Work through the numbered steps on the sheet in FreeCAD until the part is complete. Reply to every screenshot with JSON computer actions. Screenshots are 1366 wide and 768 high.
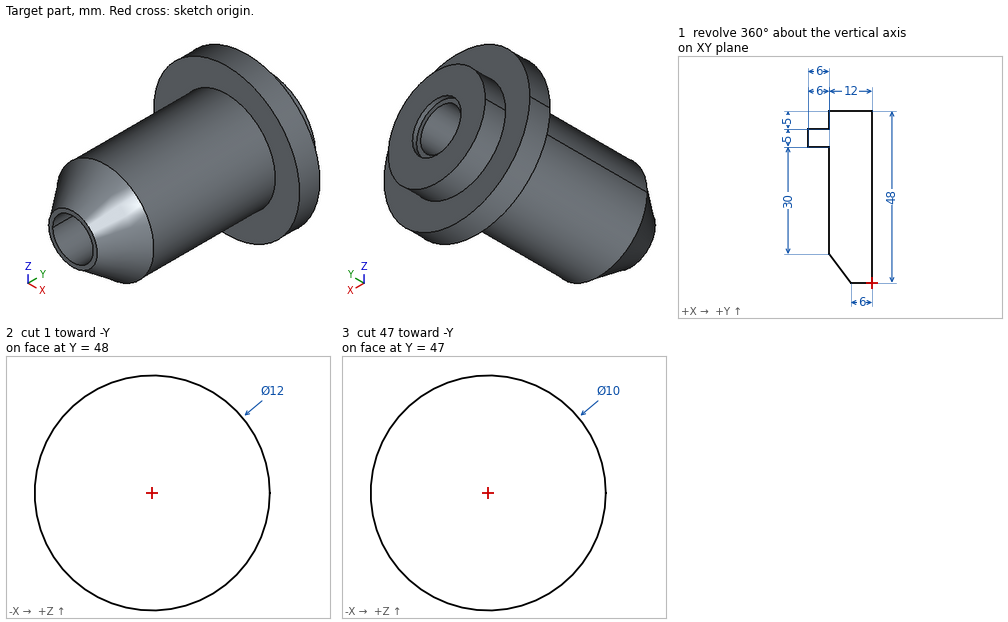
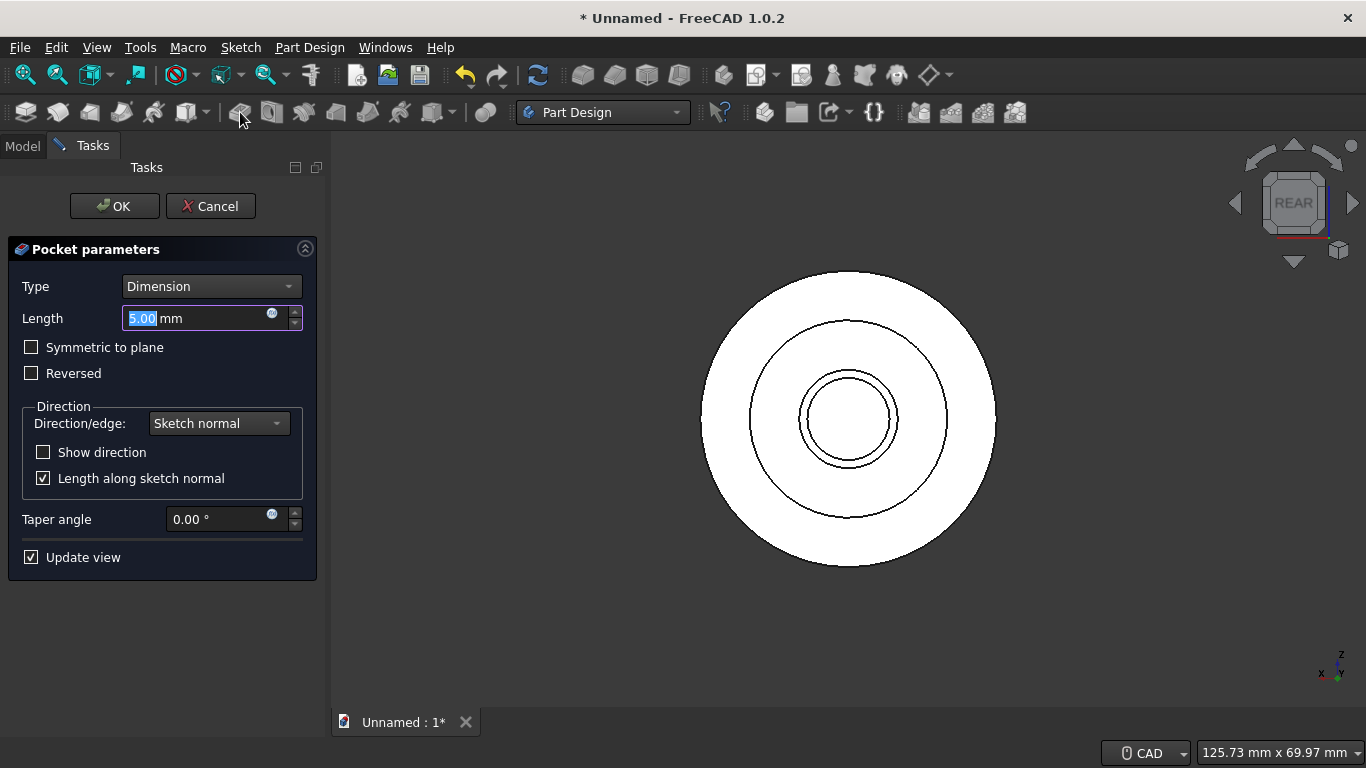
{"action": "type", "text": "47"}
{"action": "key", "text": "Tab"}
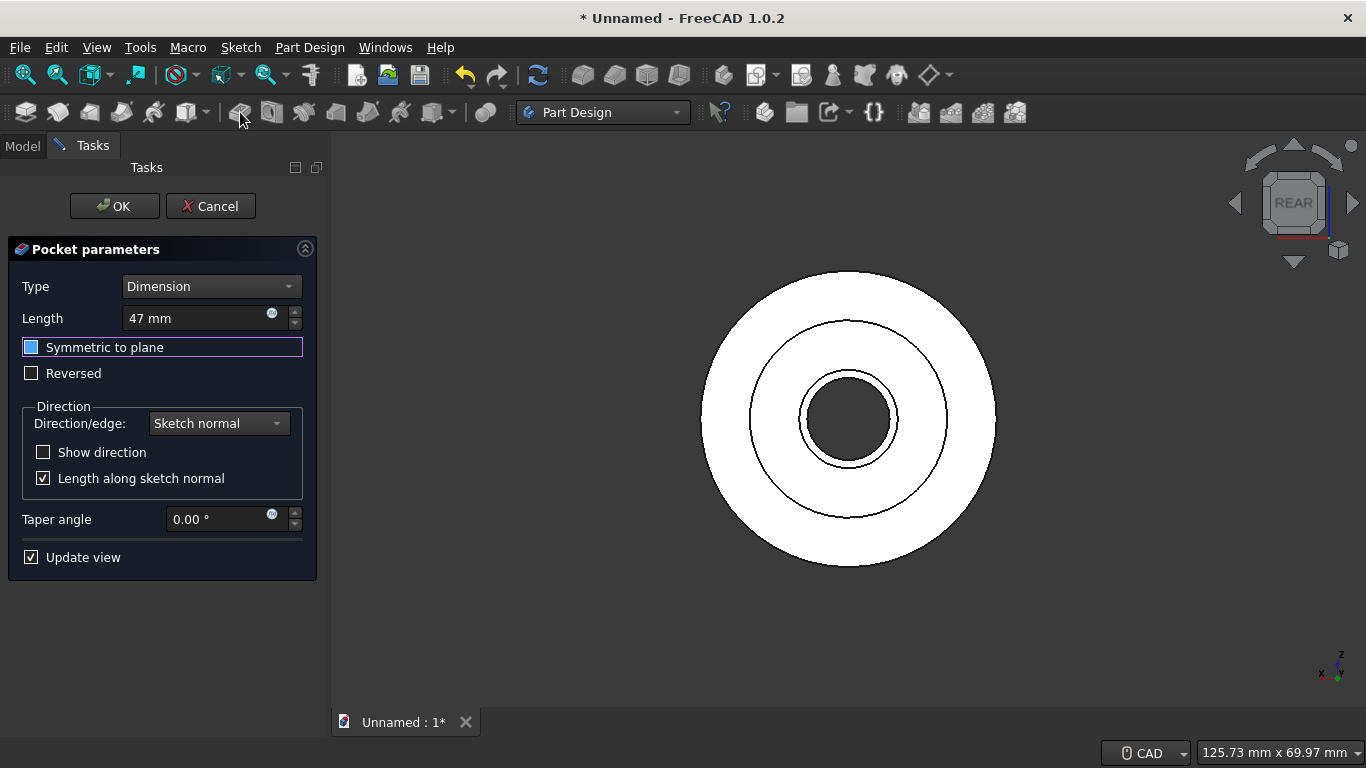
{"action": "left_click", "coordinate": [115, 206]}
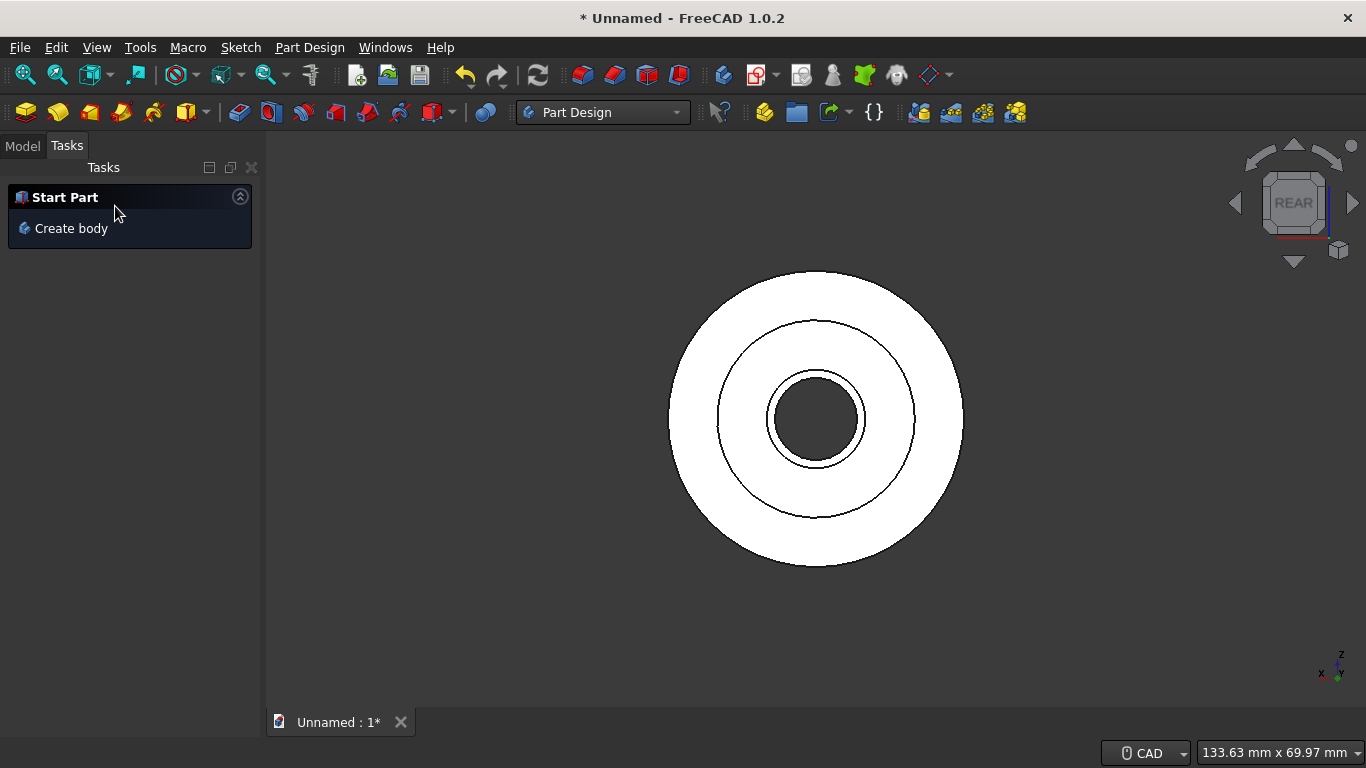
{"action": "key", "text": "0"}